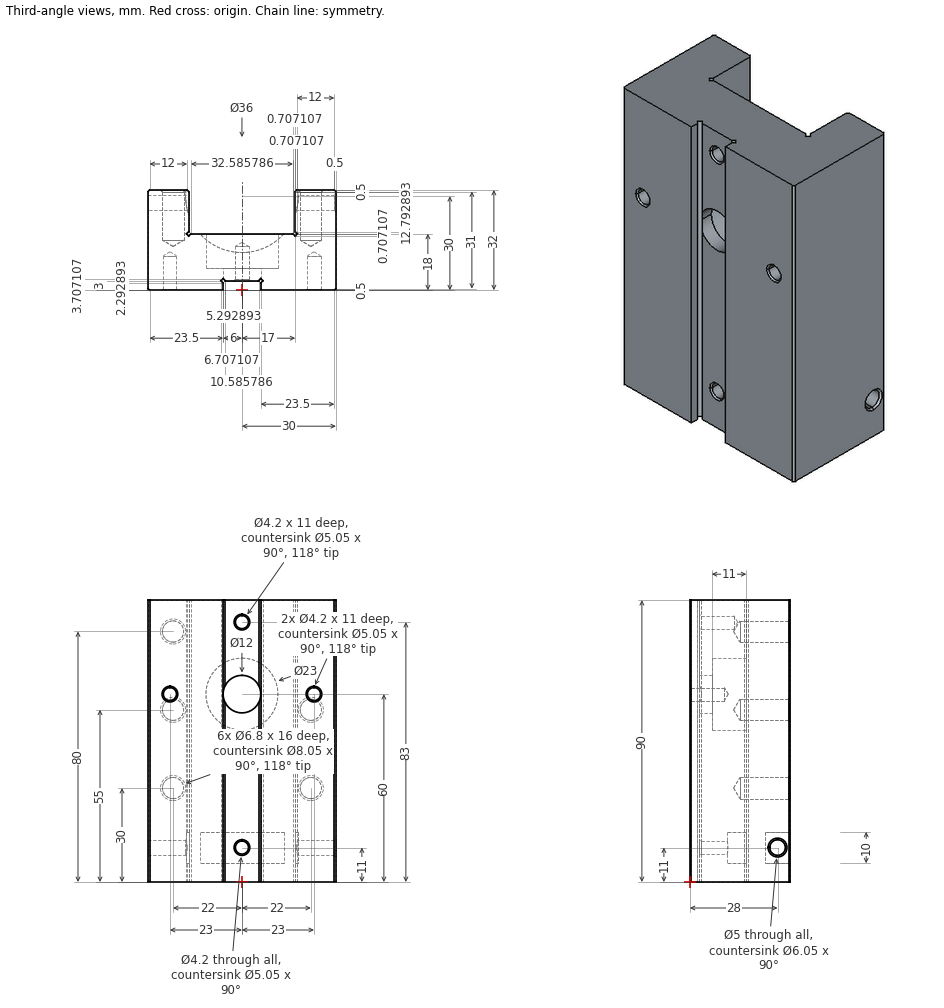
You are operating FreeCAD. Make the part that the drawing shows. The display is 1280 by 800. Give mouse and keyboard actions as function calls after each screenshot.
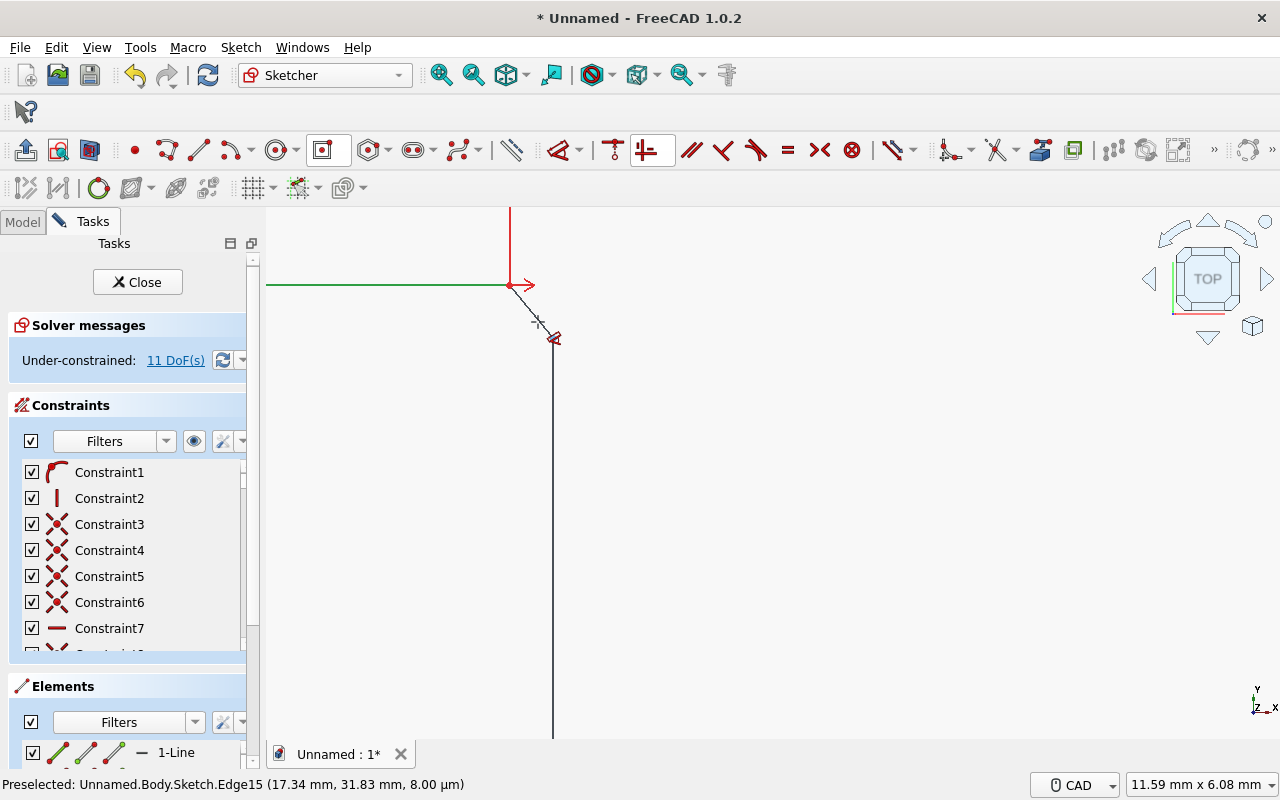
click(540, 322)
click(476, 312)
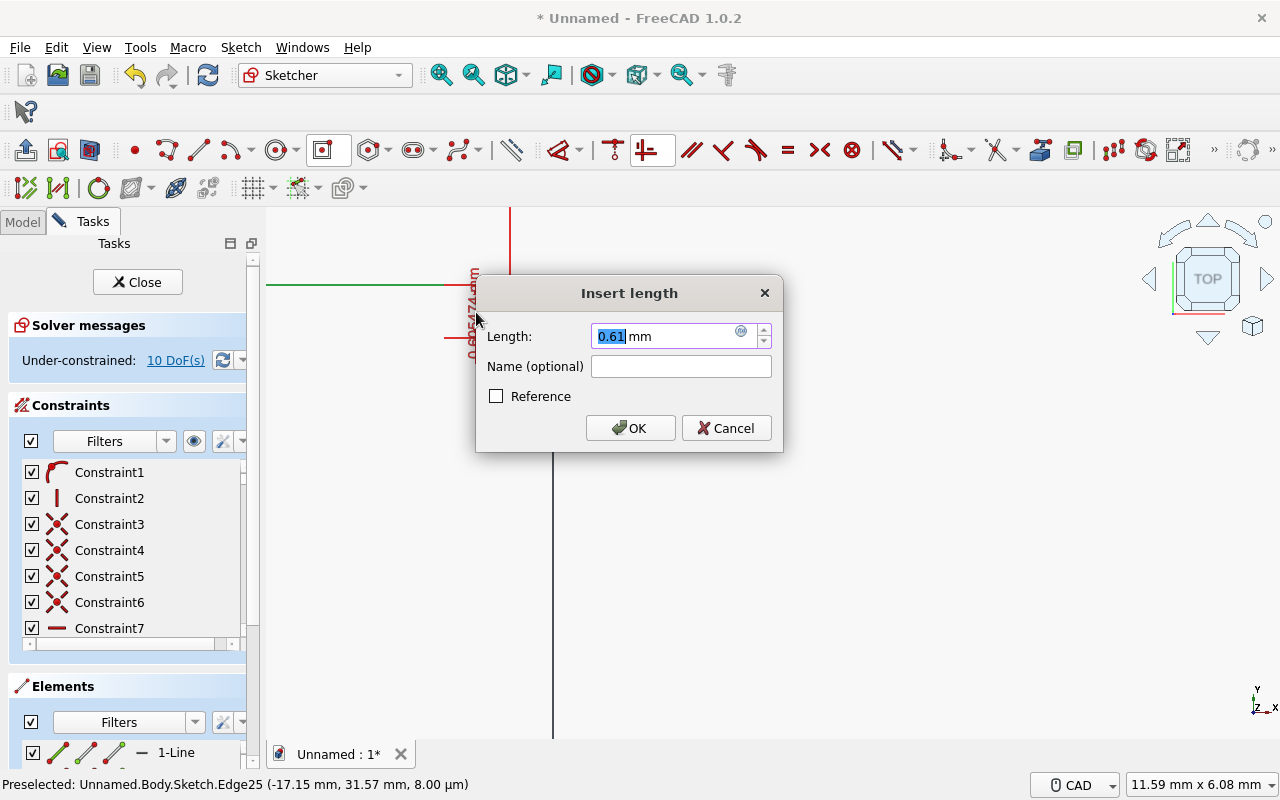
text(0.5)
key(Return)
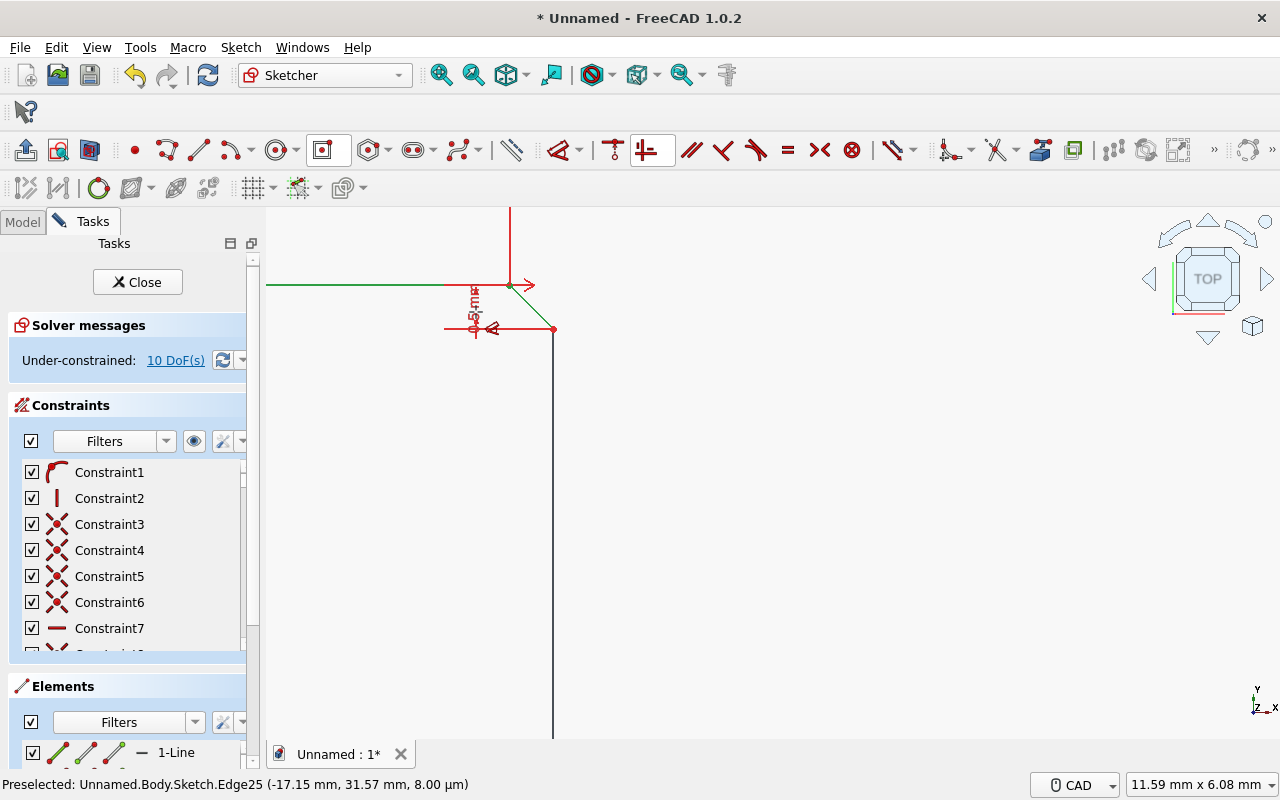
scroll(538, 322, down, 11)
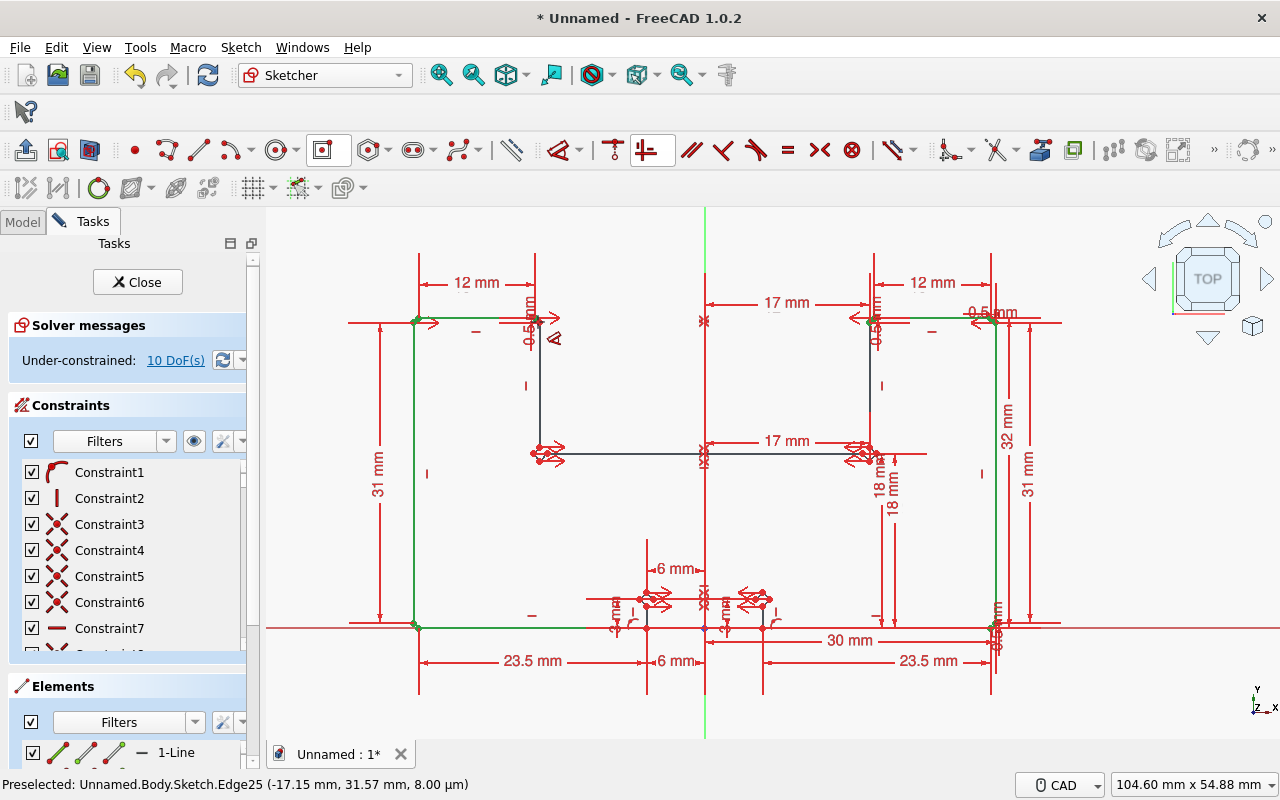
scroll(647, 622, up, 4)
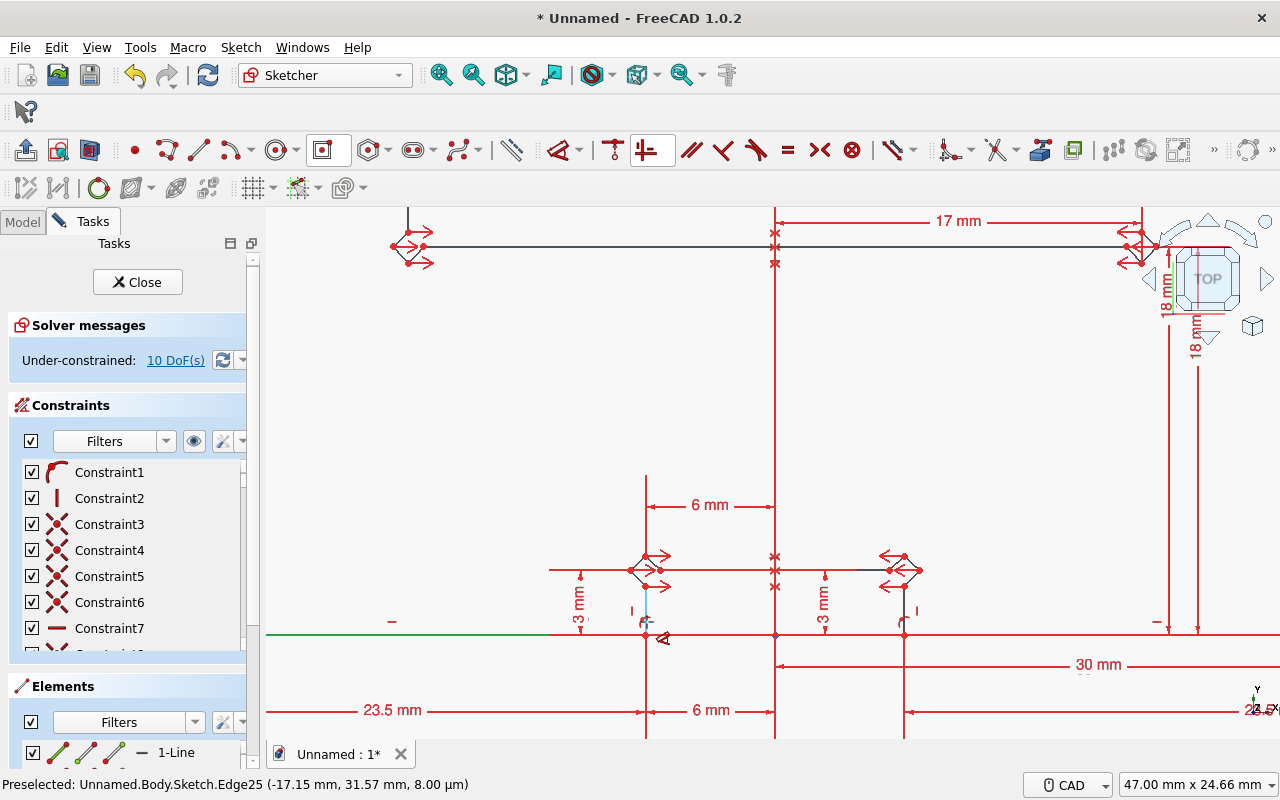
click(646, 621)
click(680, 611)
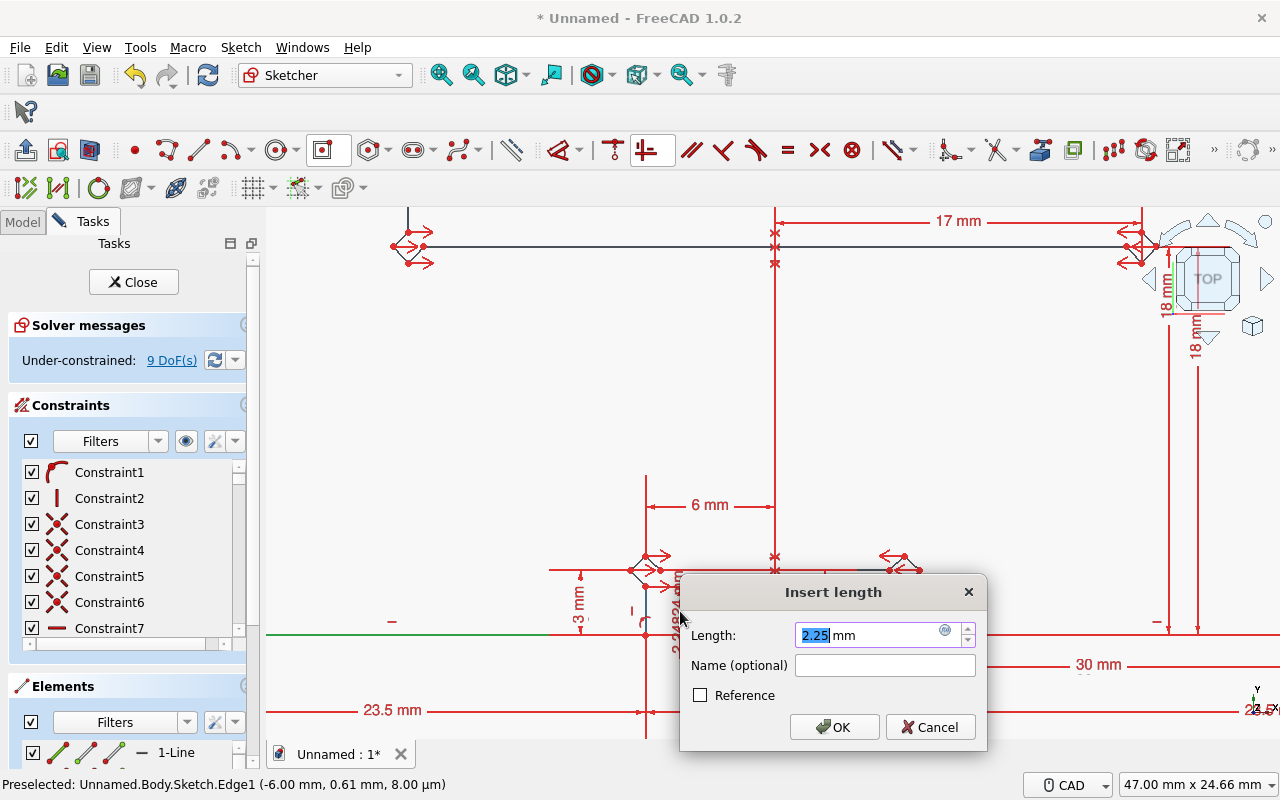
text(2.292893)
key(Return)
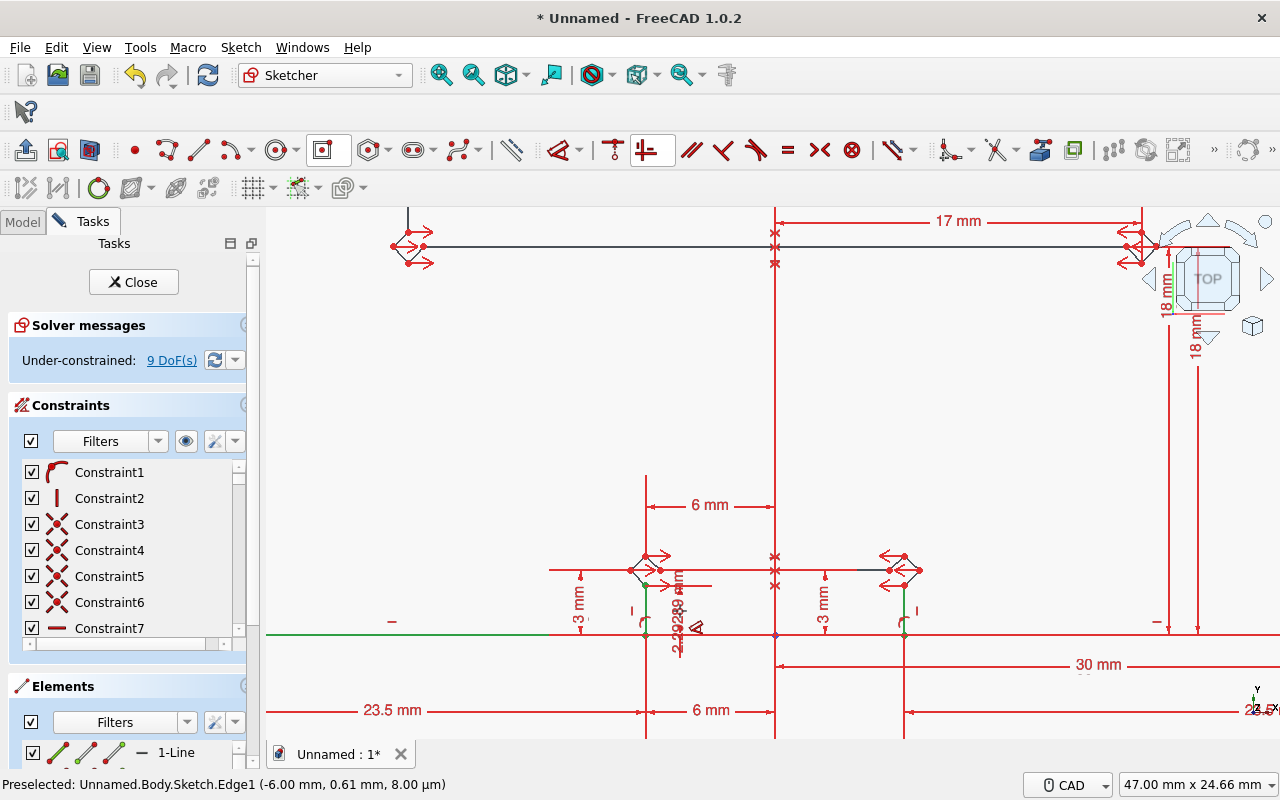
click(729, 570)
click(722, 536)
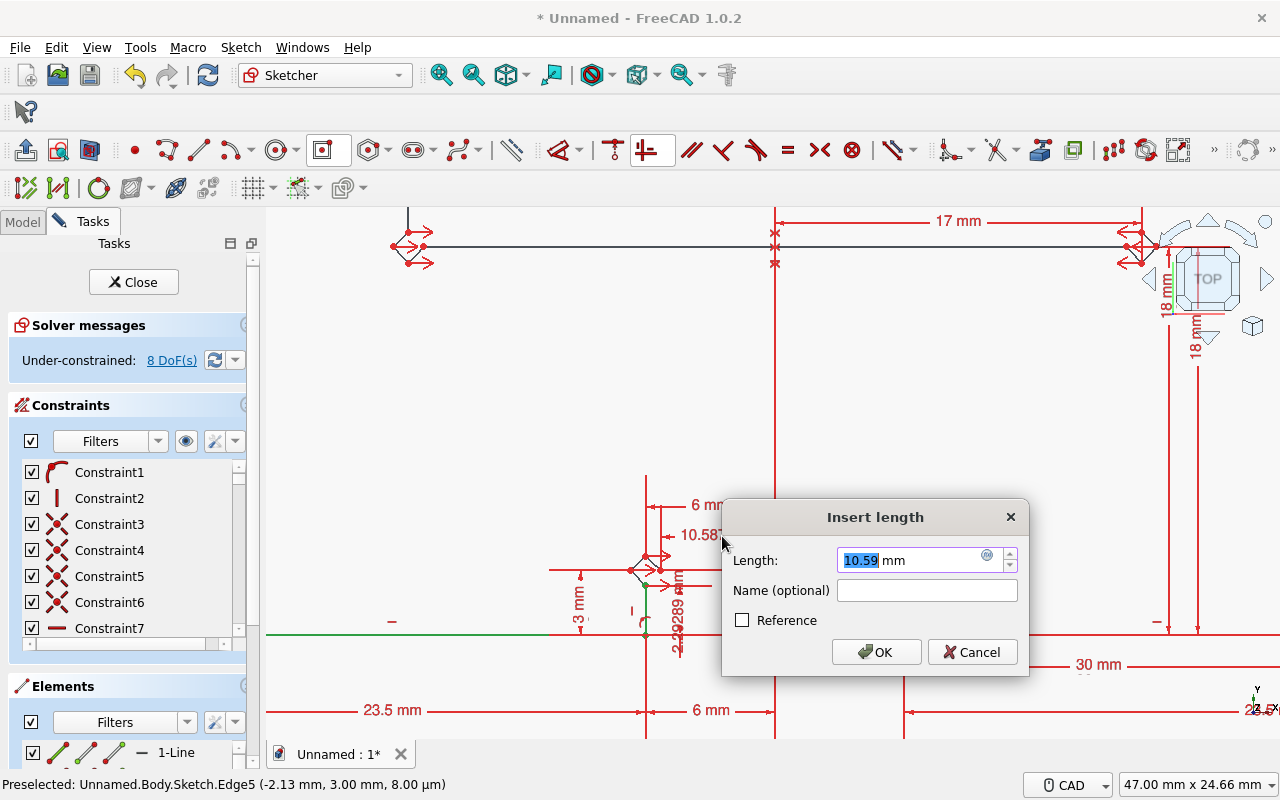
text(10.585786)
key(Return)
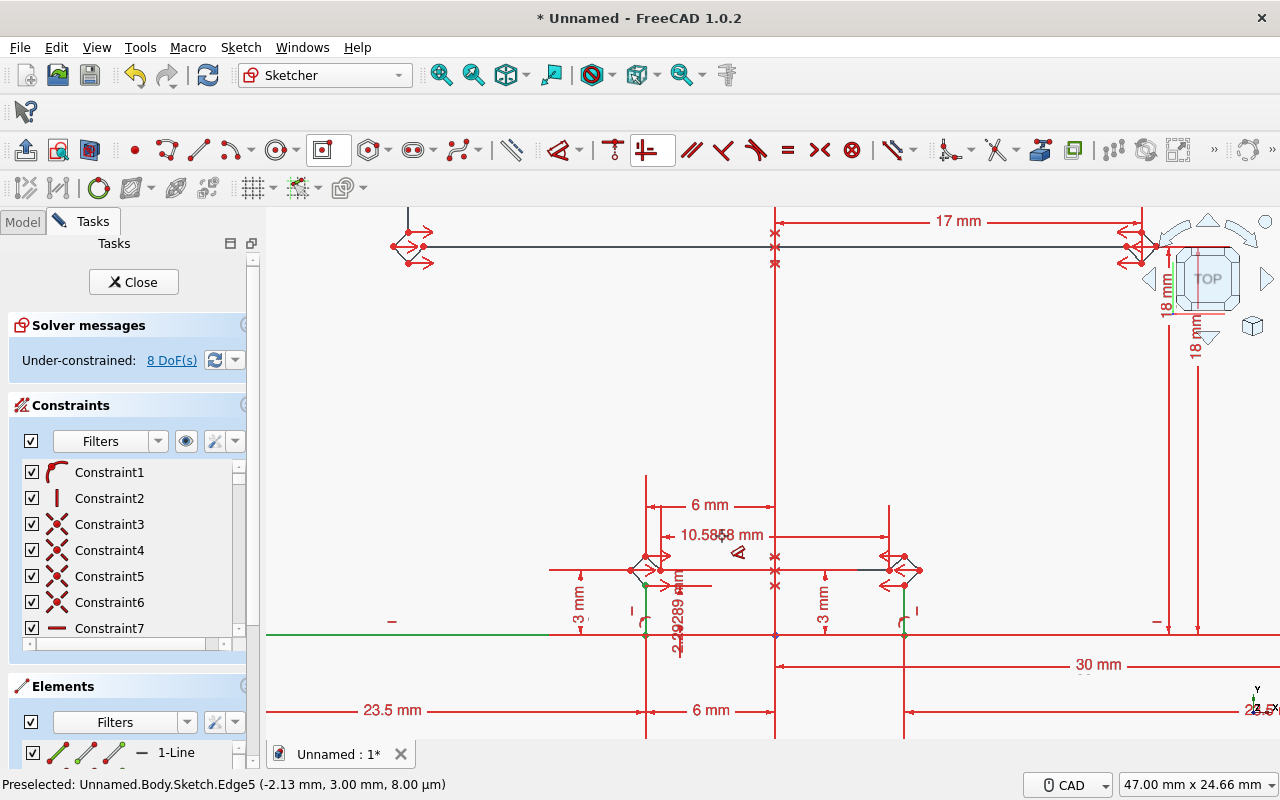
scroll(647, 622, down, 4)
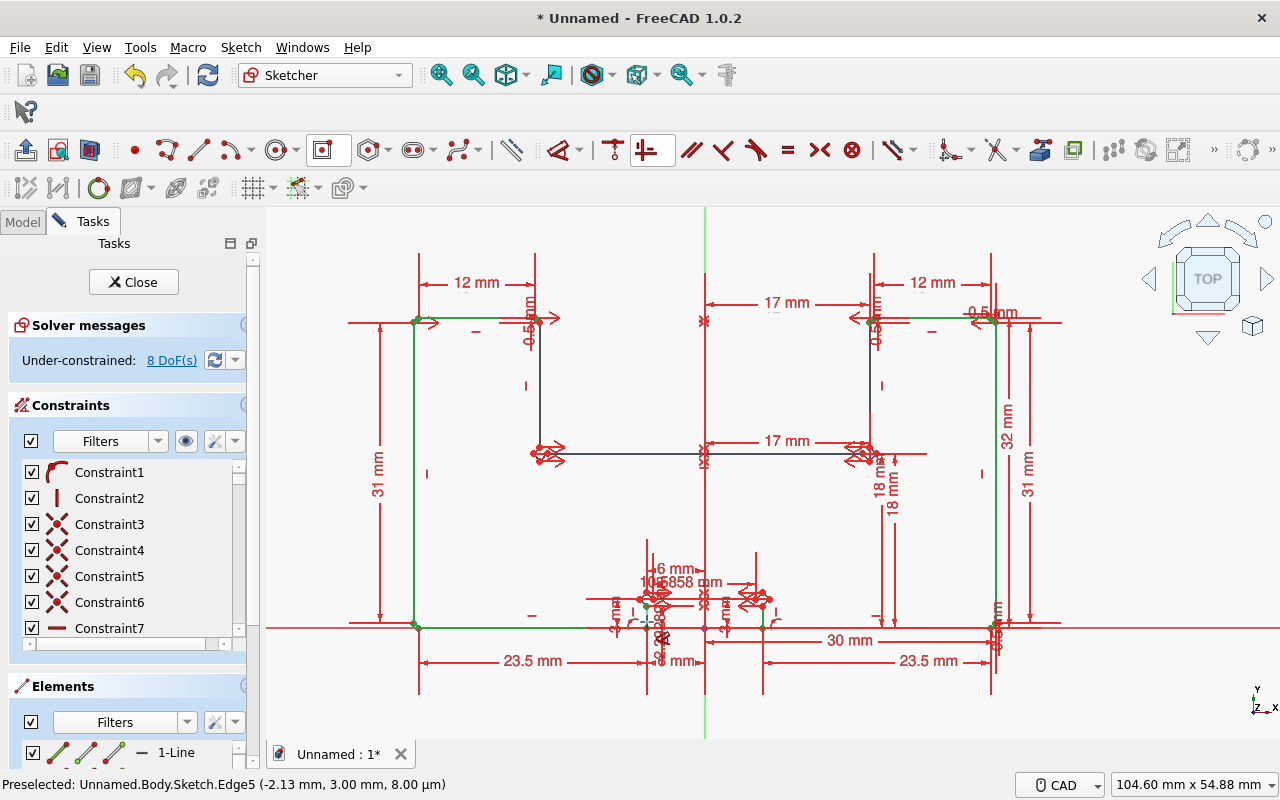
click(870, 360)
click(904, 385)